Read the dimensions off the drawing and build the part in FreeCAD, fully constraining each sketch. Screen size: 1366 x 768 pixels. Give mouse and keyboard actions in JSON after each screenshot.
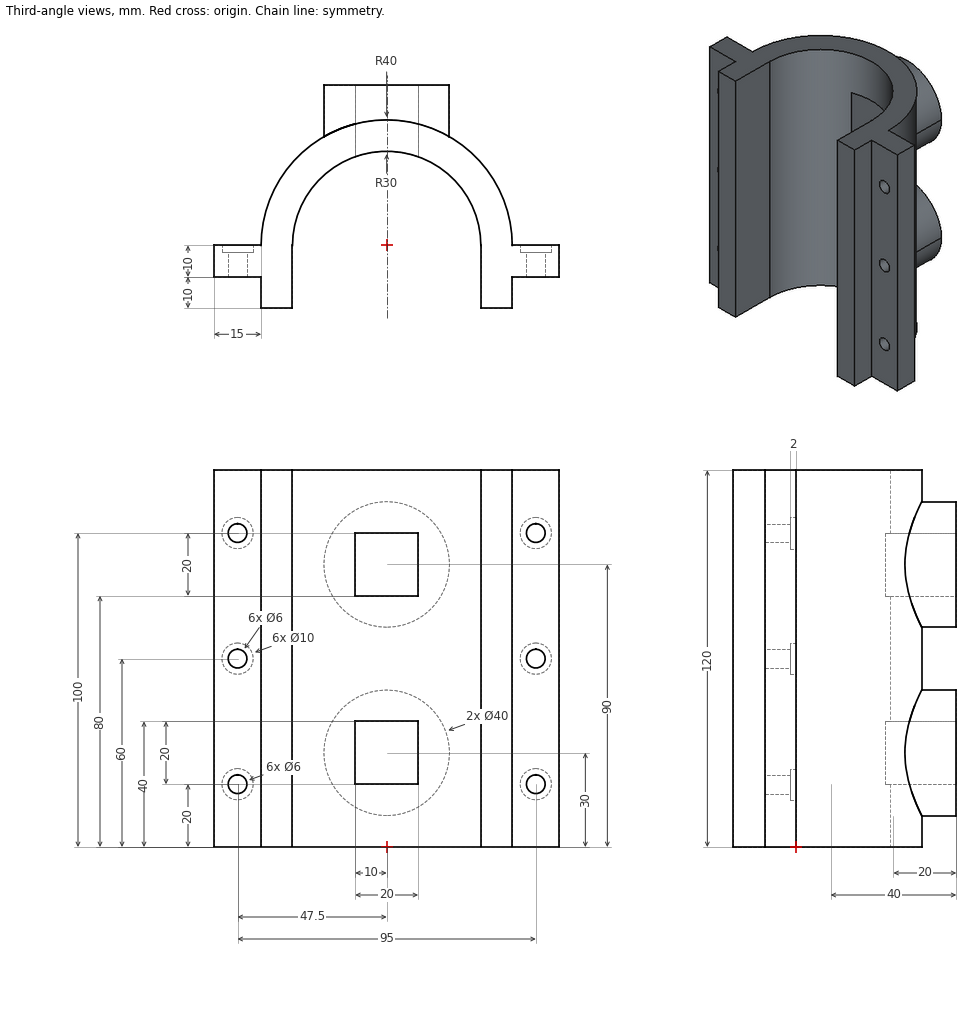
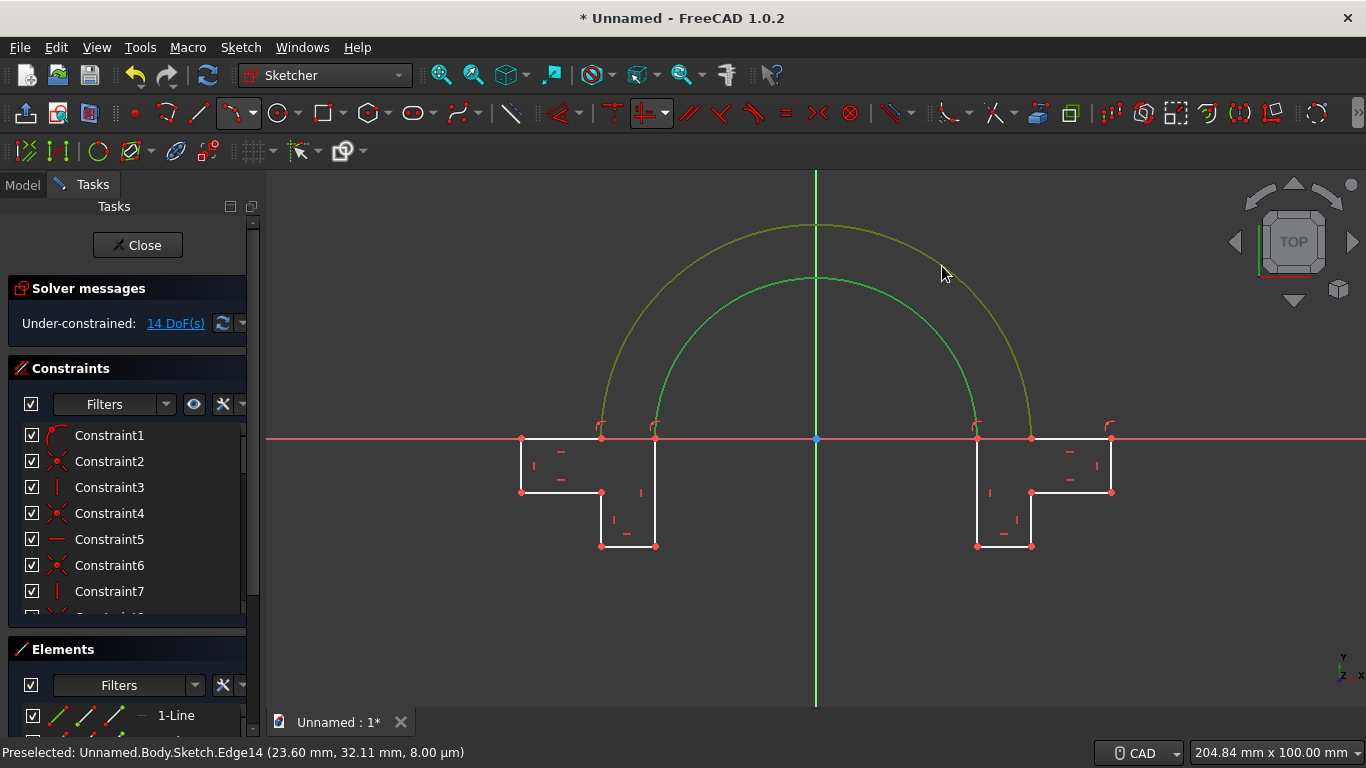
{"action": "left_click", "coordinate": [614, 114]}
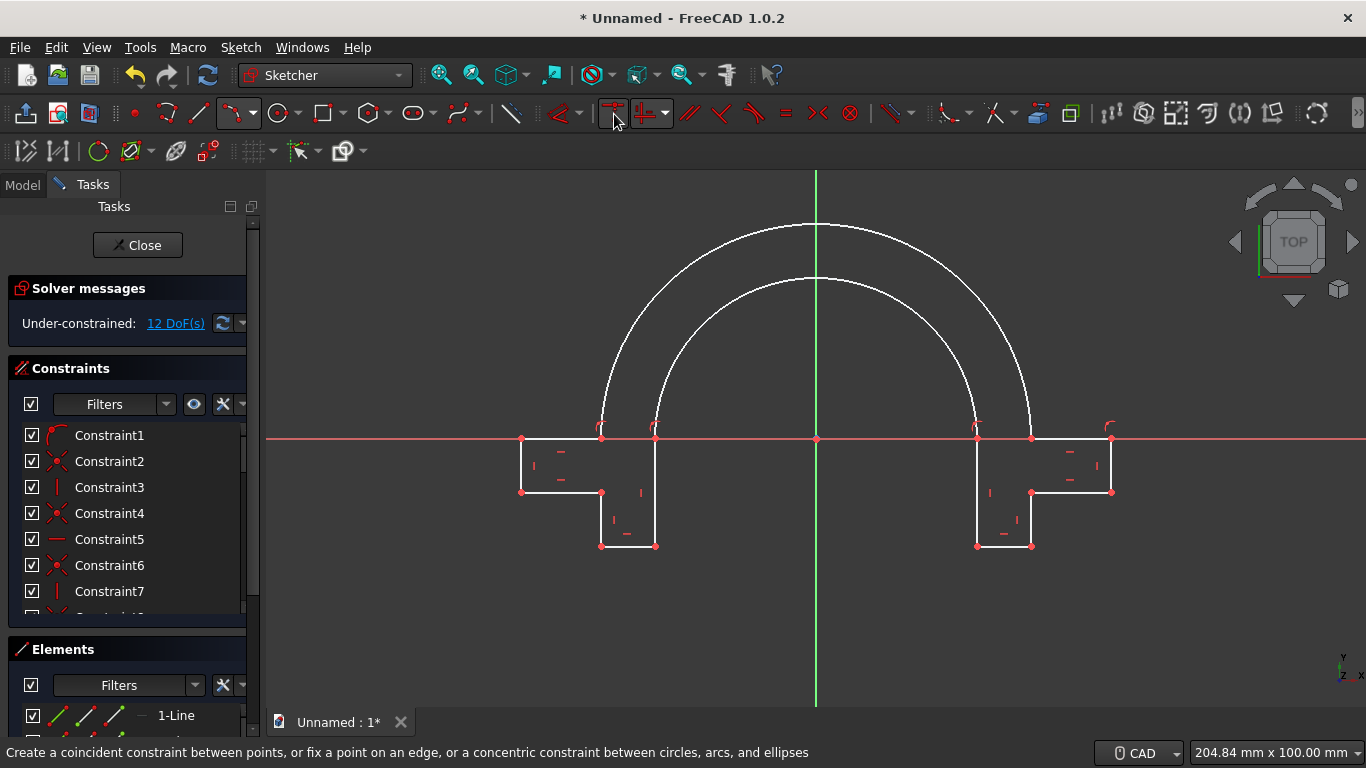
{"action": "left_click_drag", "start_coordinate": [806, 428], "coordinate": [826, 449]}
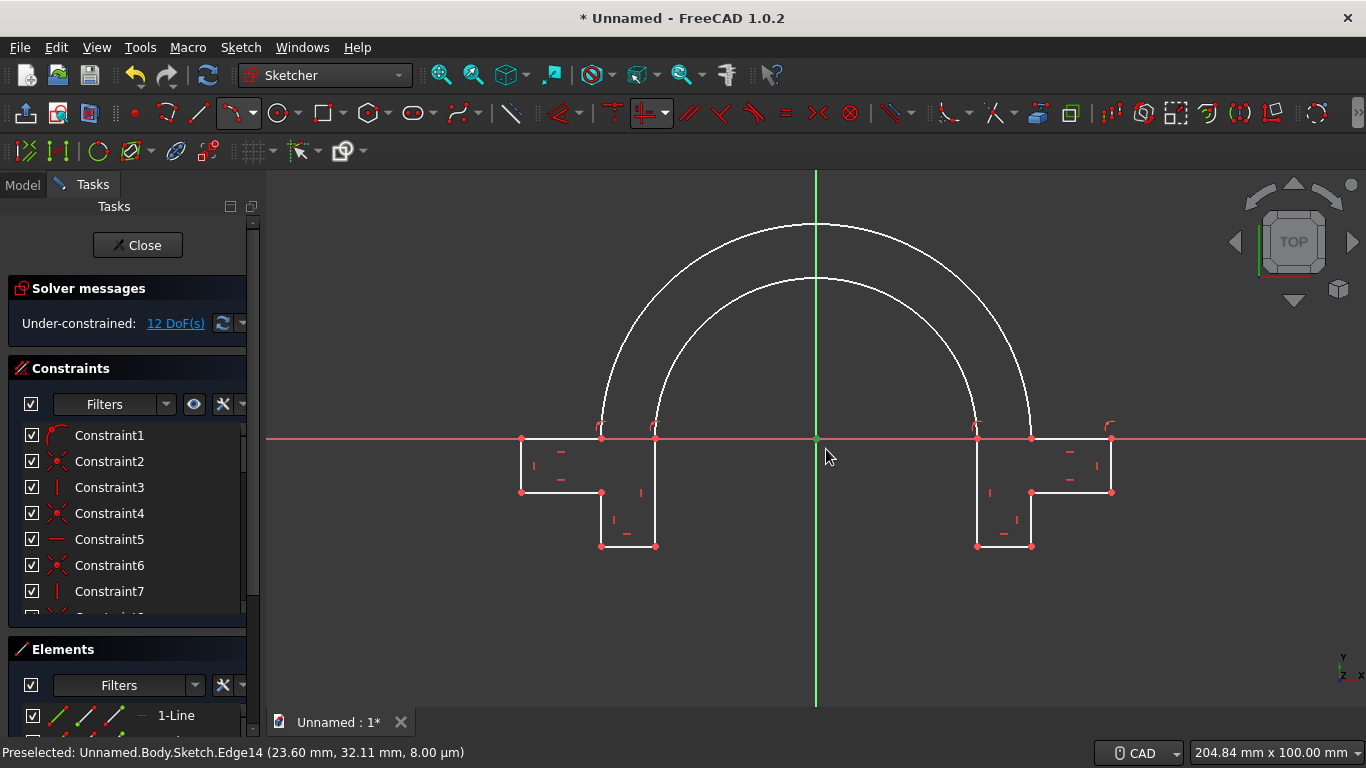
{"action": "left_click", "coordinate": [614, 114]}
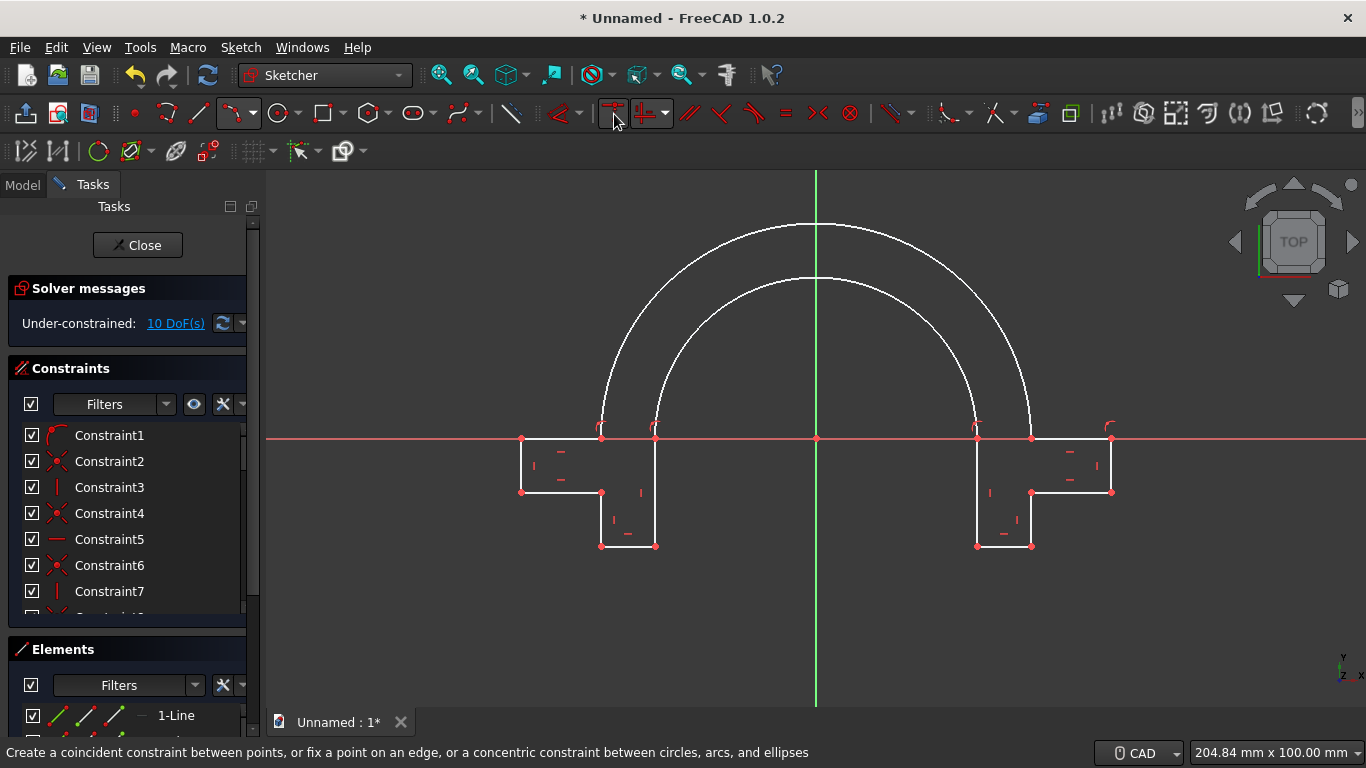
{"action": "left_click", "coordinate": [601, 547]}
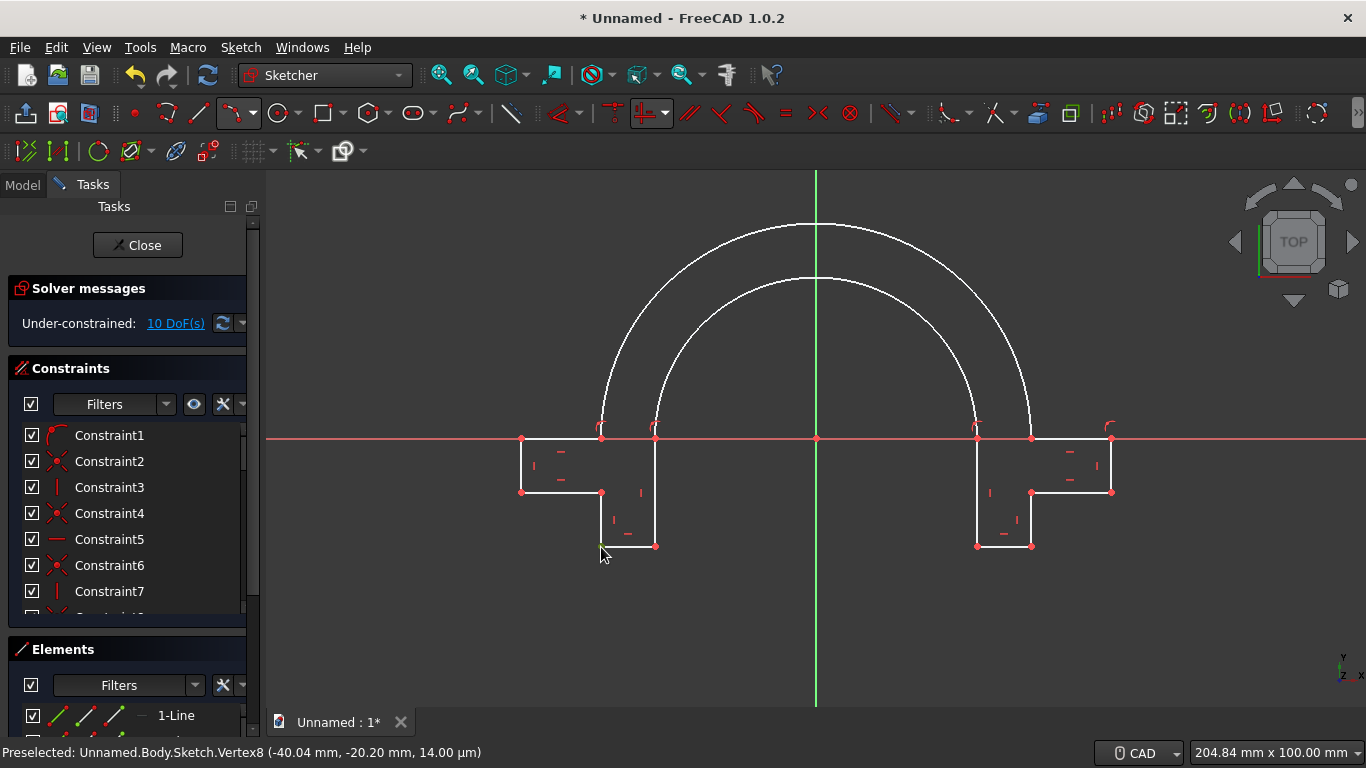
{"action": "left_click", "coordinate": [1031, 547]}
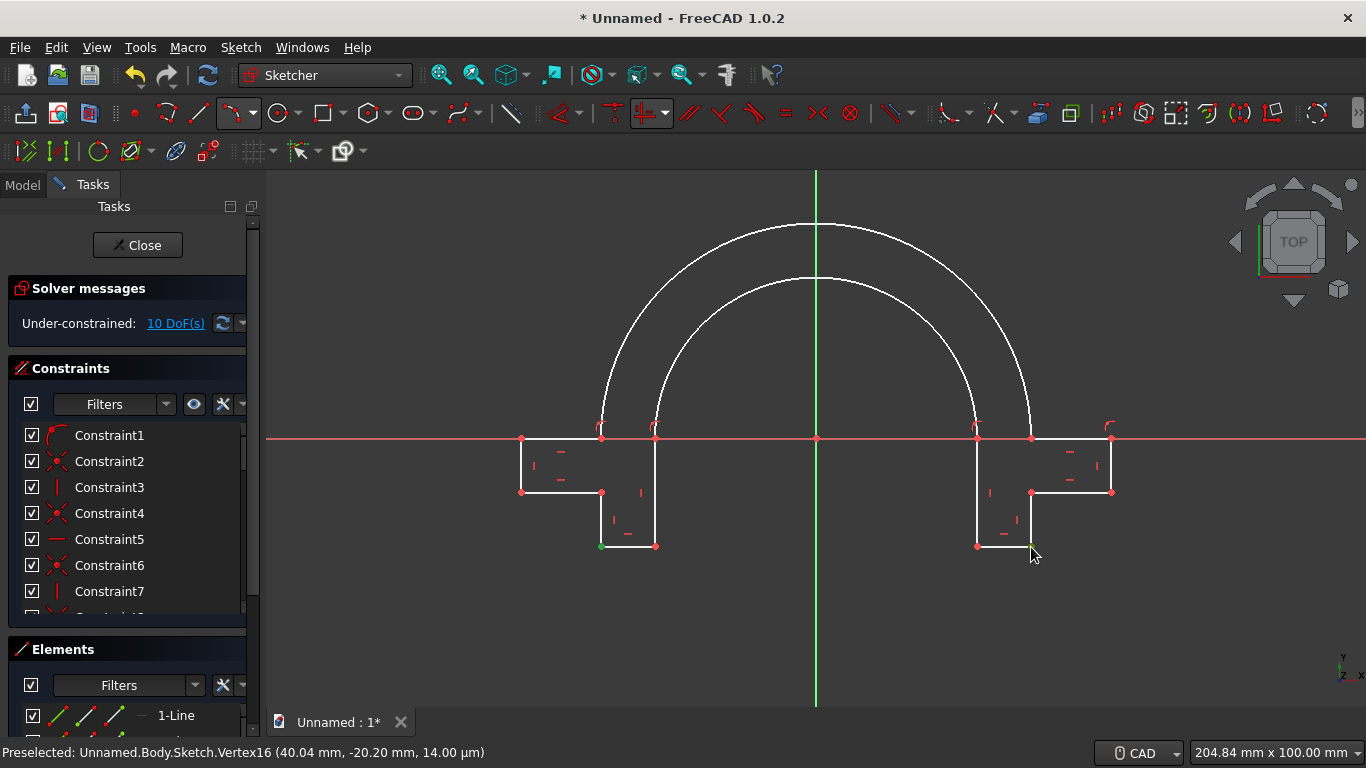
{"action": "left_click", "coordinate": [816, 645]}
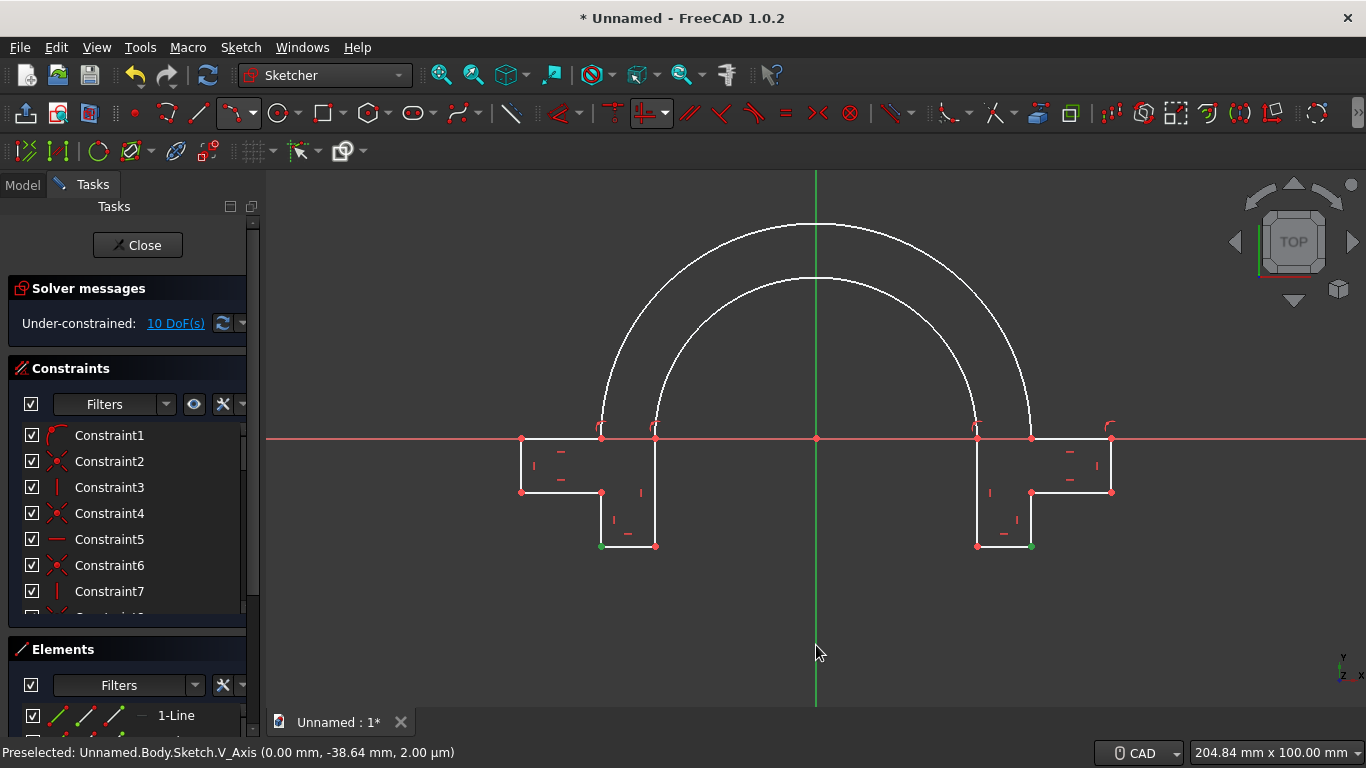
{"action": "left_click", "coordinate": [818, 114]}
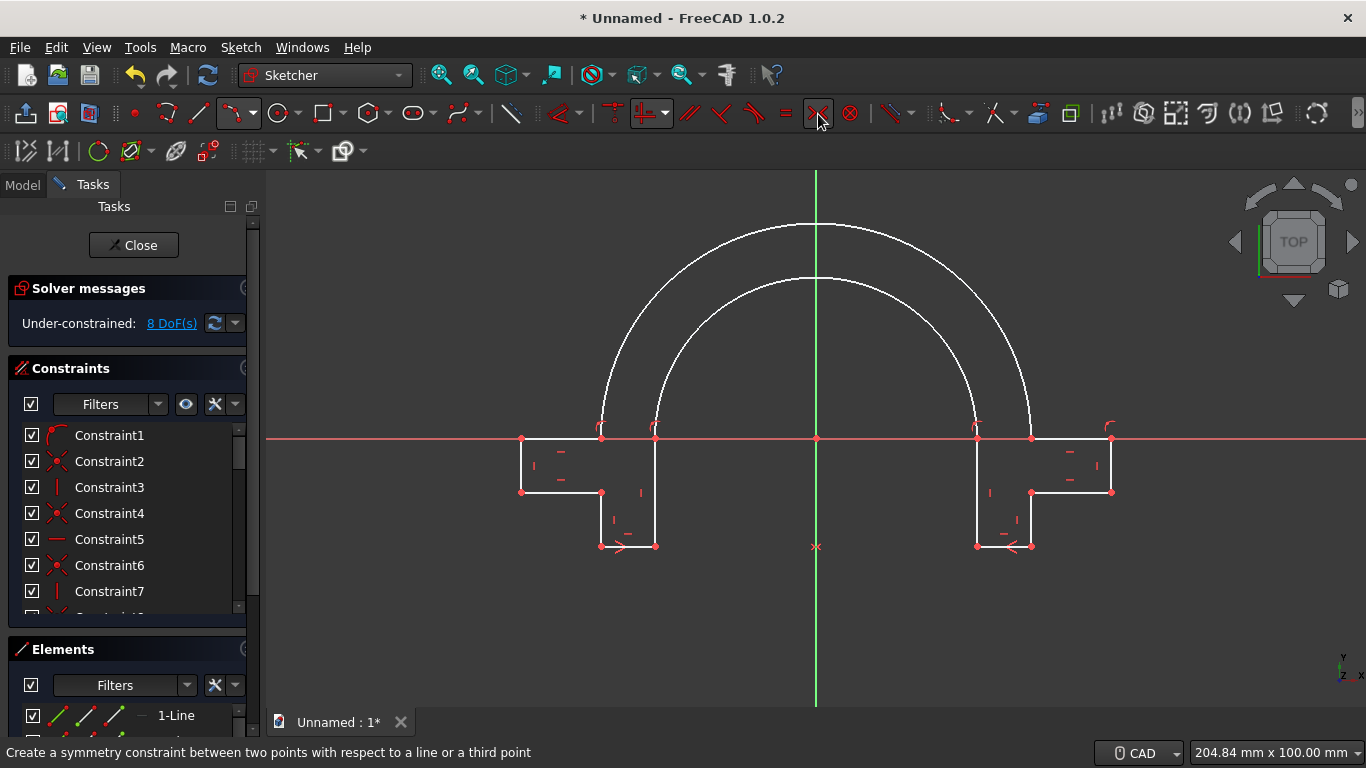
{"action": "left_click", "coordinate": [521, 493]}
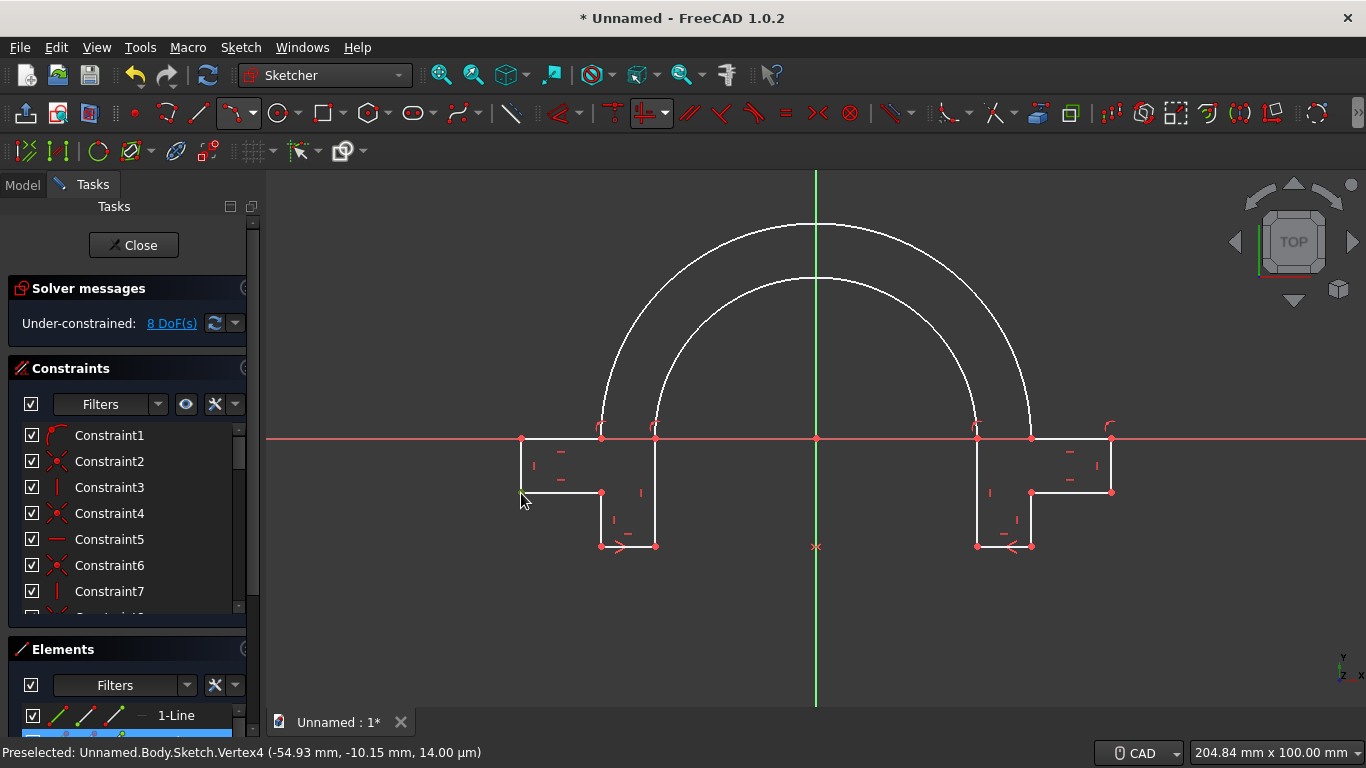
{"action": "left_click", "coordinate": [1111, 493]}